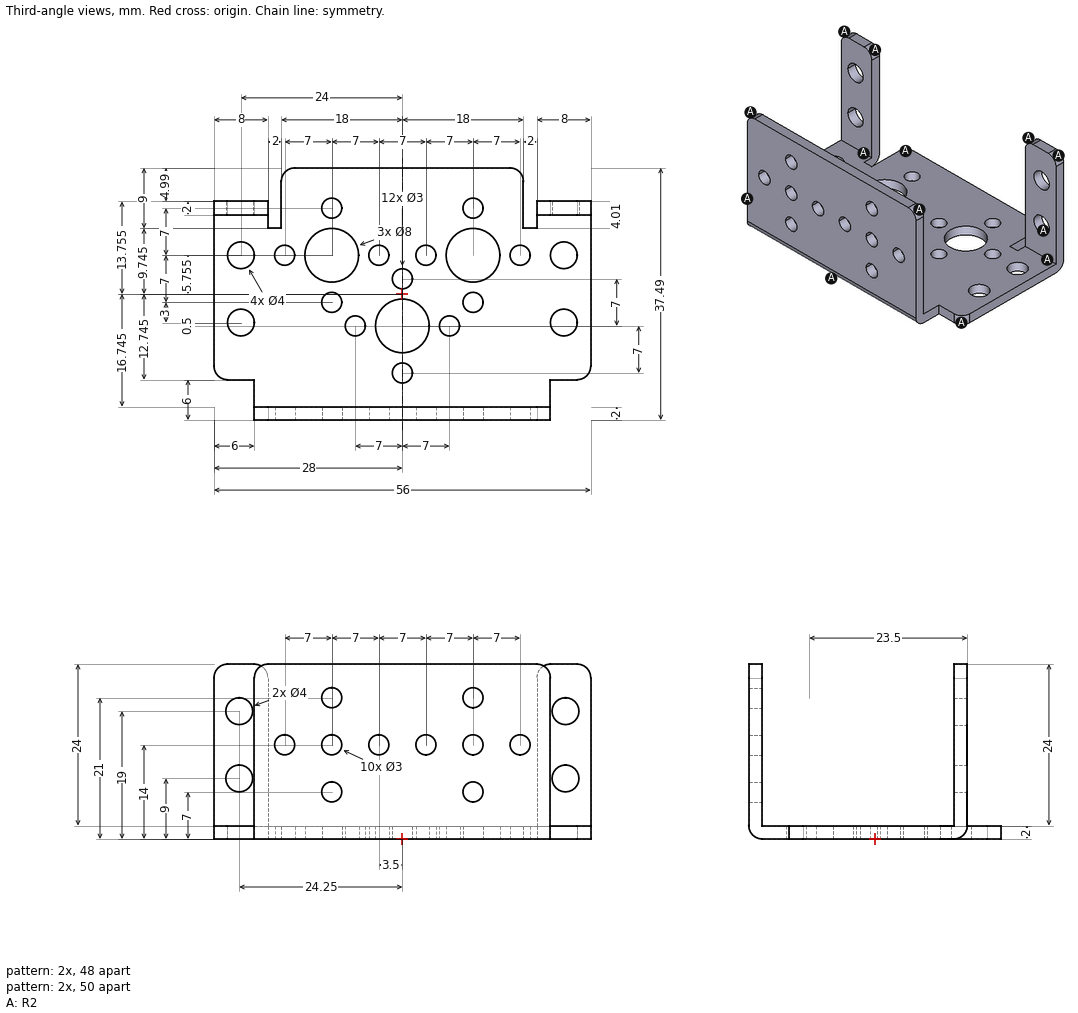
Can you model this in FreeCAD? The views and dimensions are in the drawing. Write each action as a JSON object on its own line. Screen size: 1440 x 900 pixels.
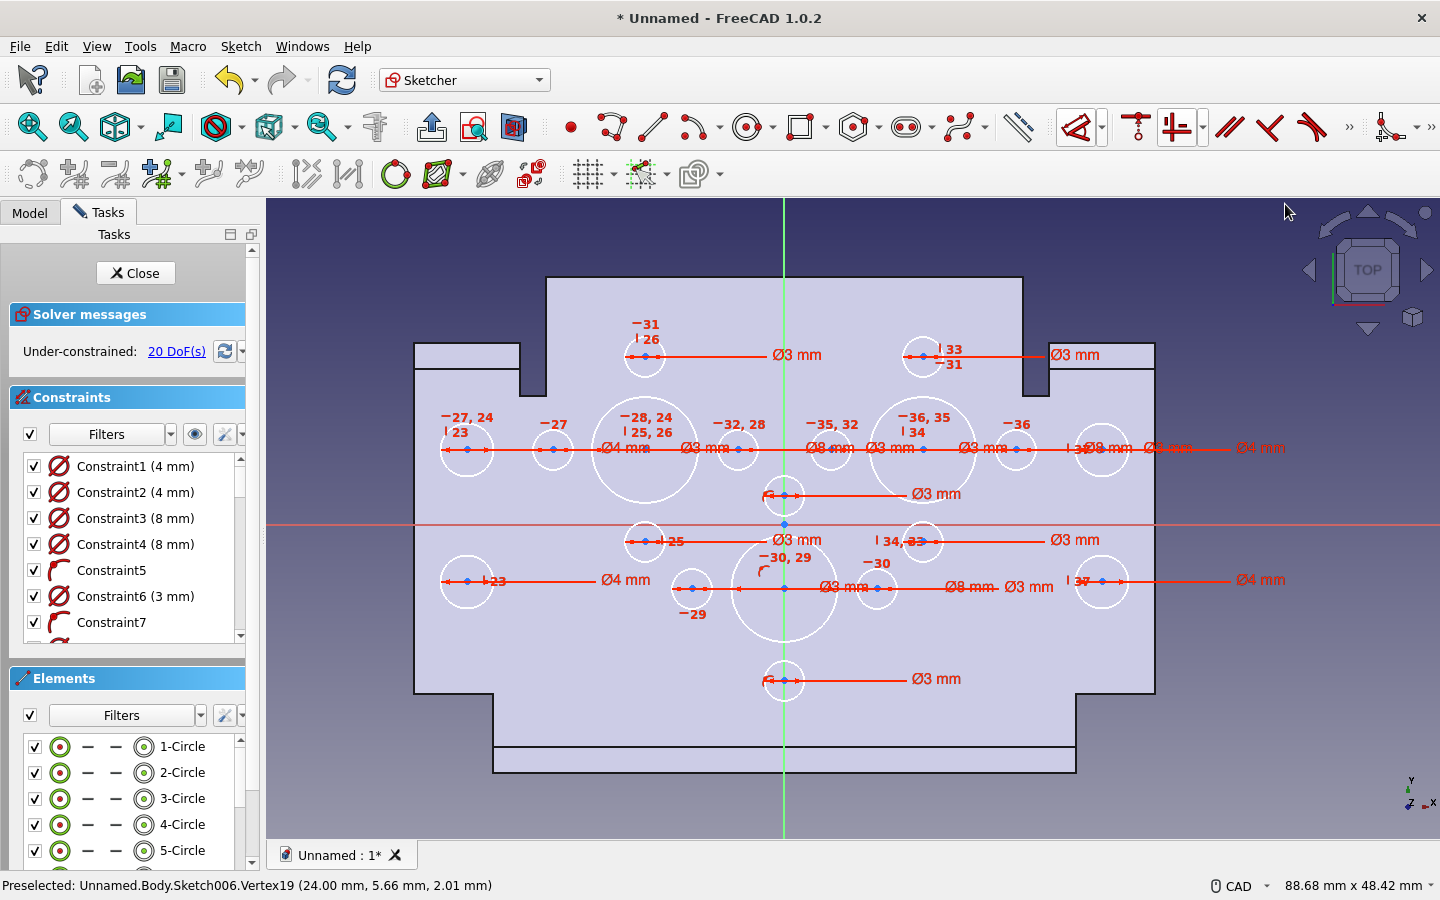
{"action": "left_click", "coordinate": [1016, 450]}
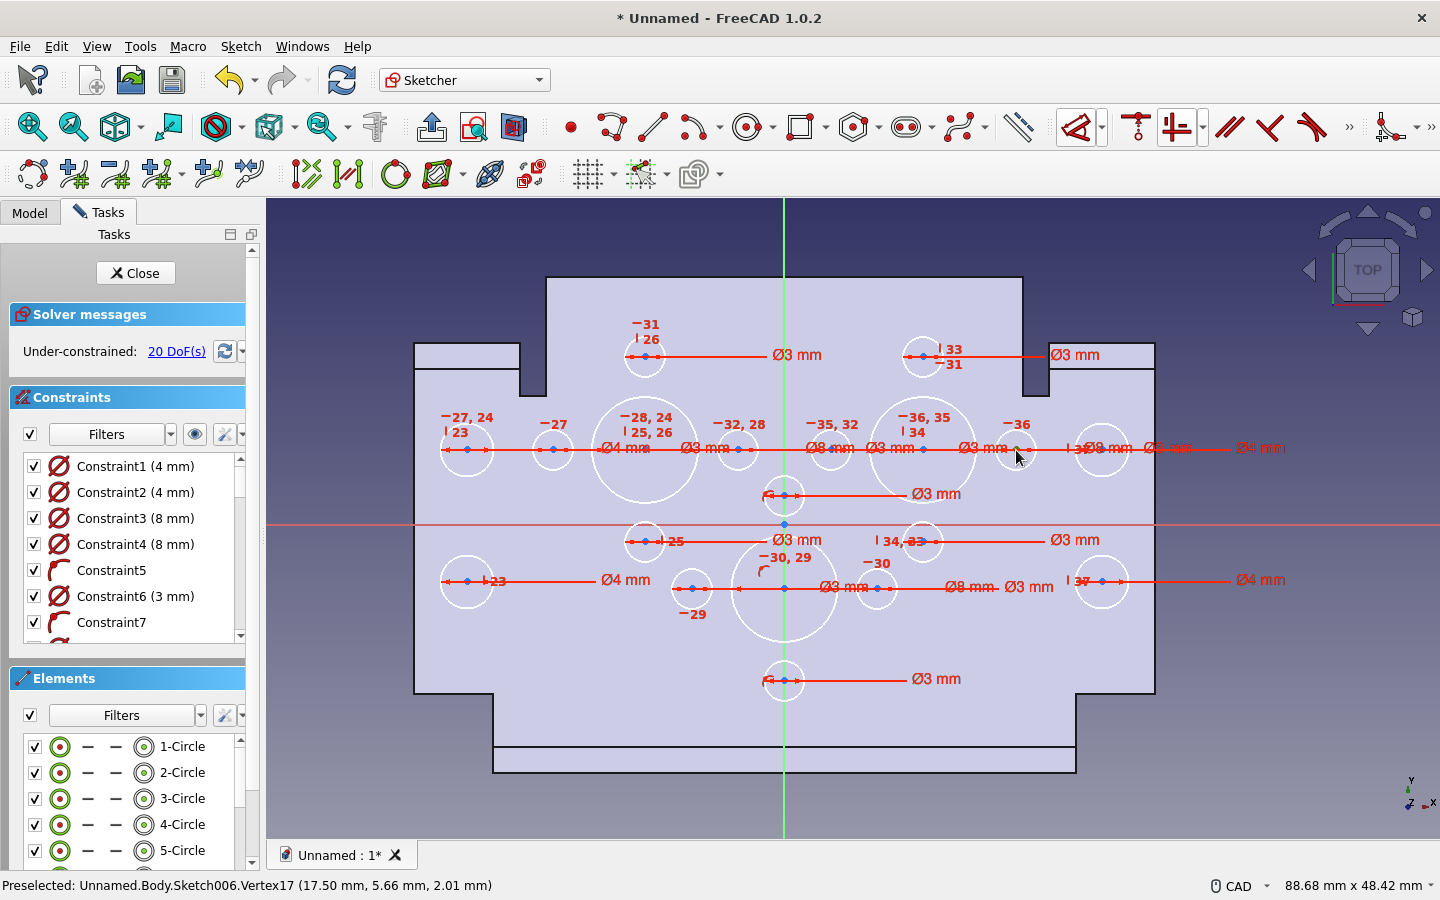
{"action": "left_click", "coordinate": [1102, 450]}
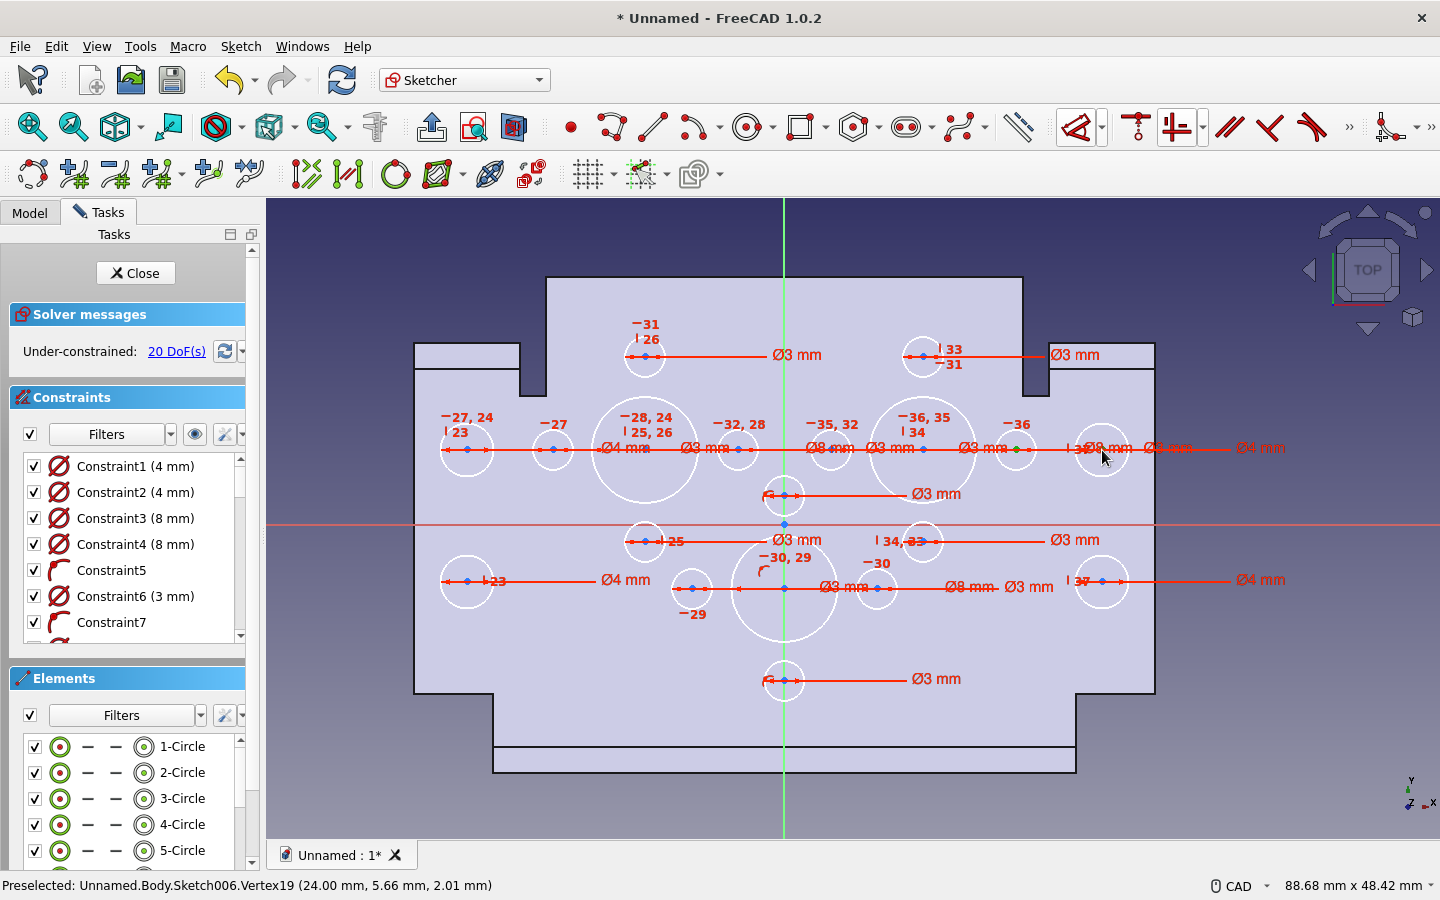
{"action": "left_click", "coordinate": [1202, 128]}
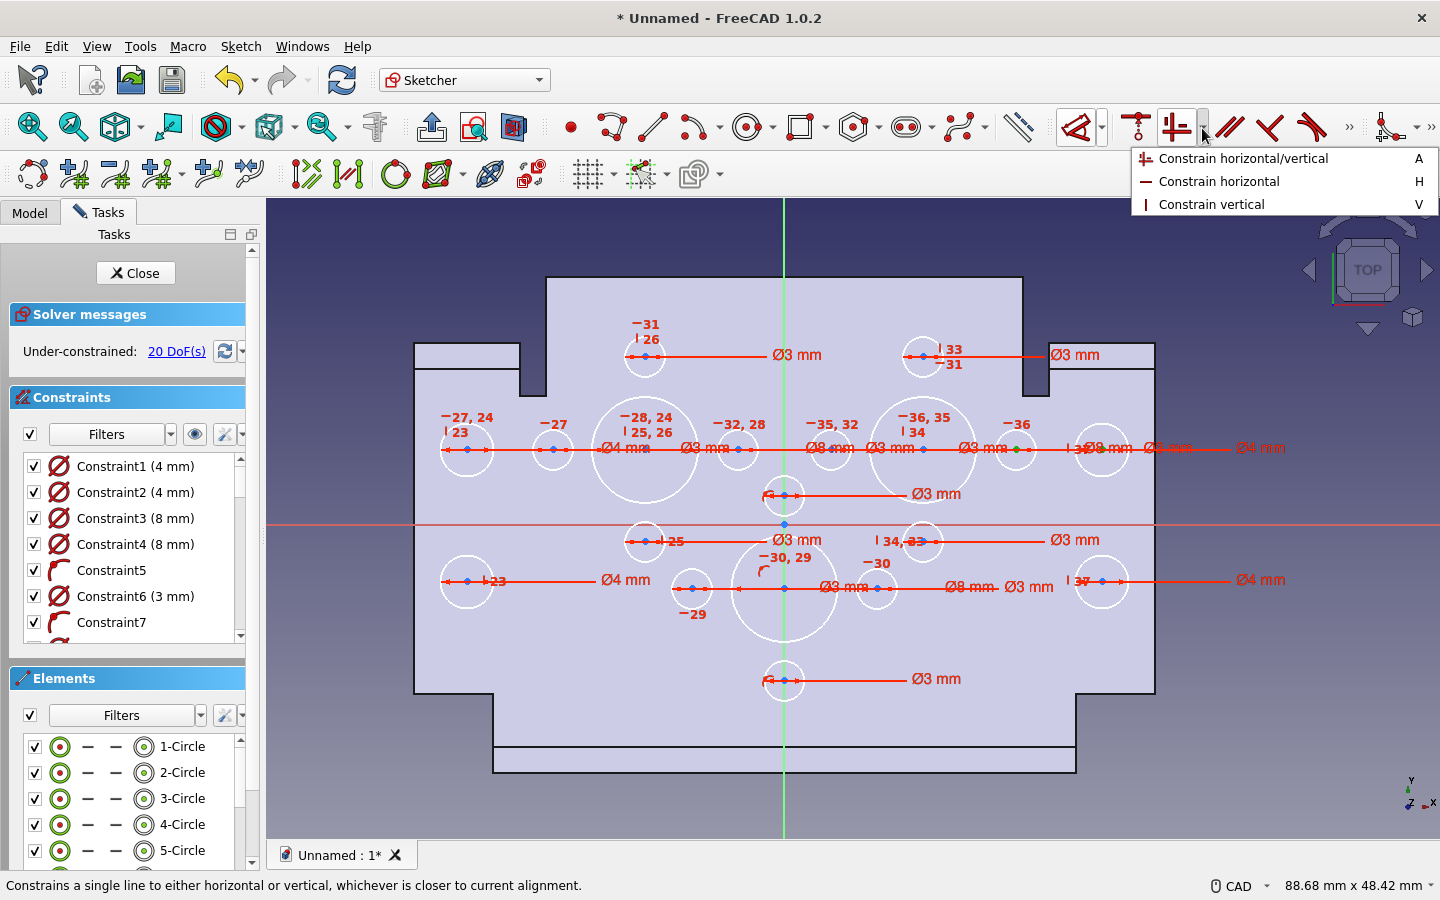
{"action": "left_click", "coordinate": [1285, 182]}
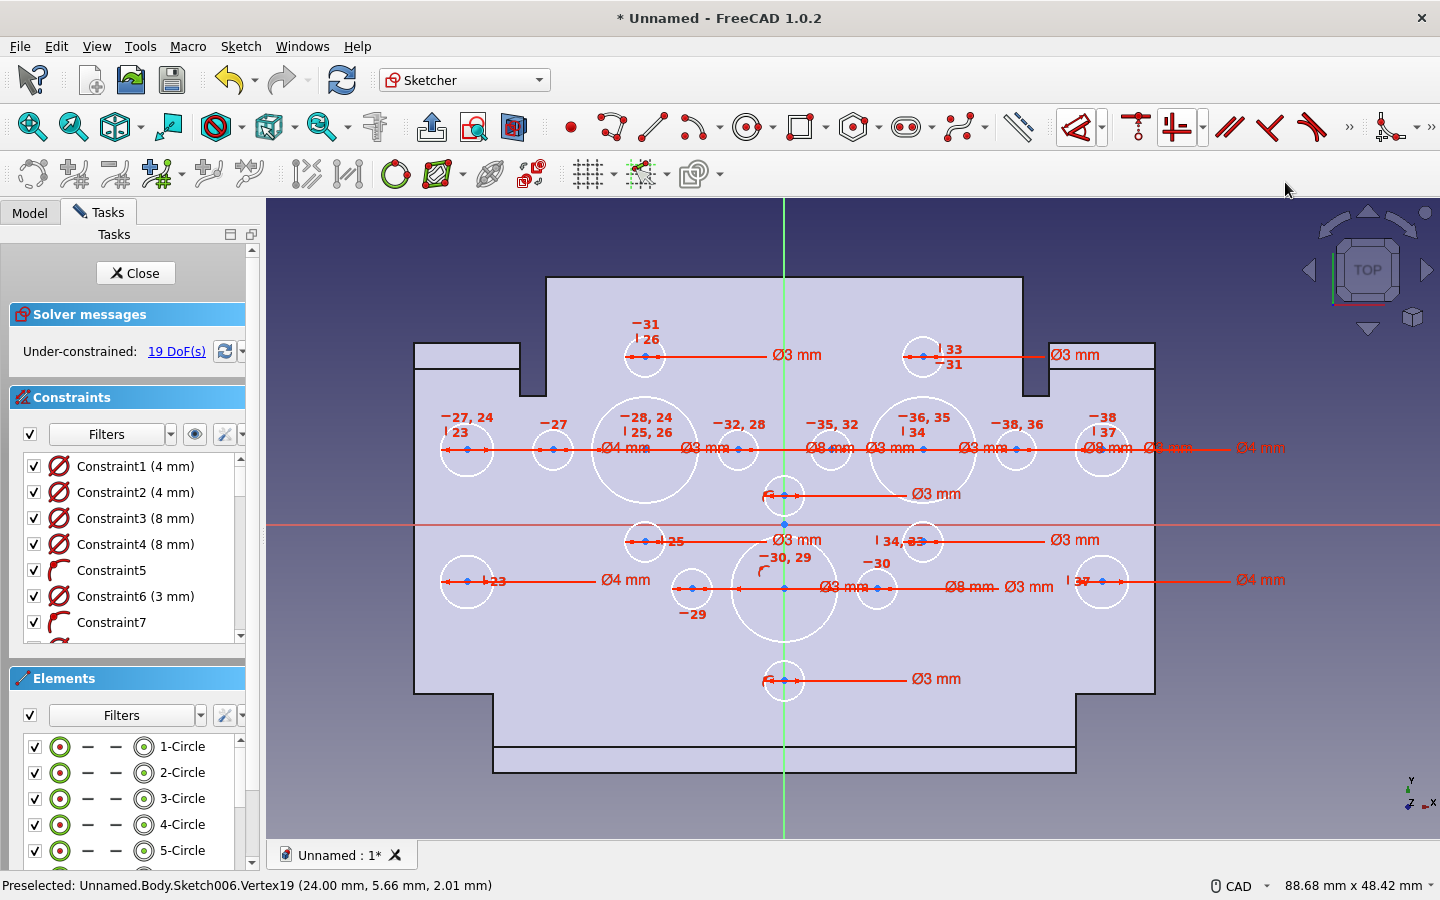
{"action": "left_click", "coordinate": [645, 542]}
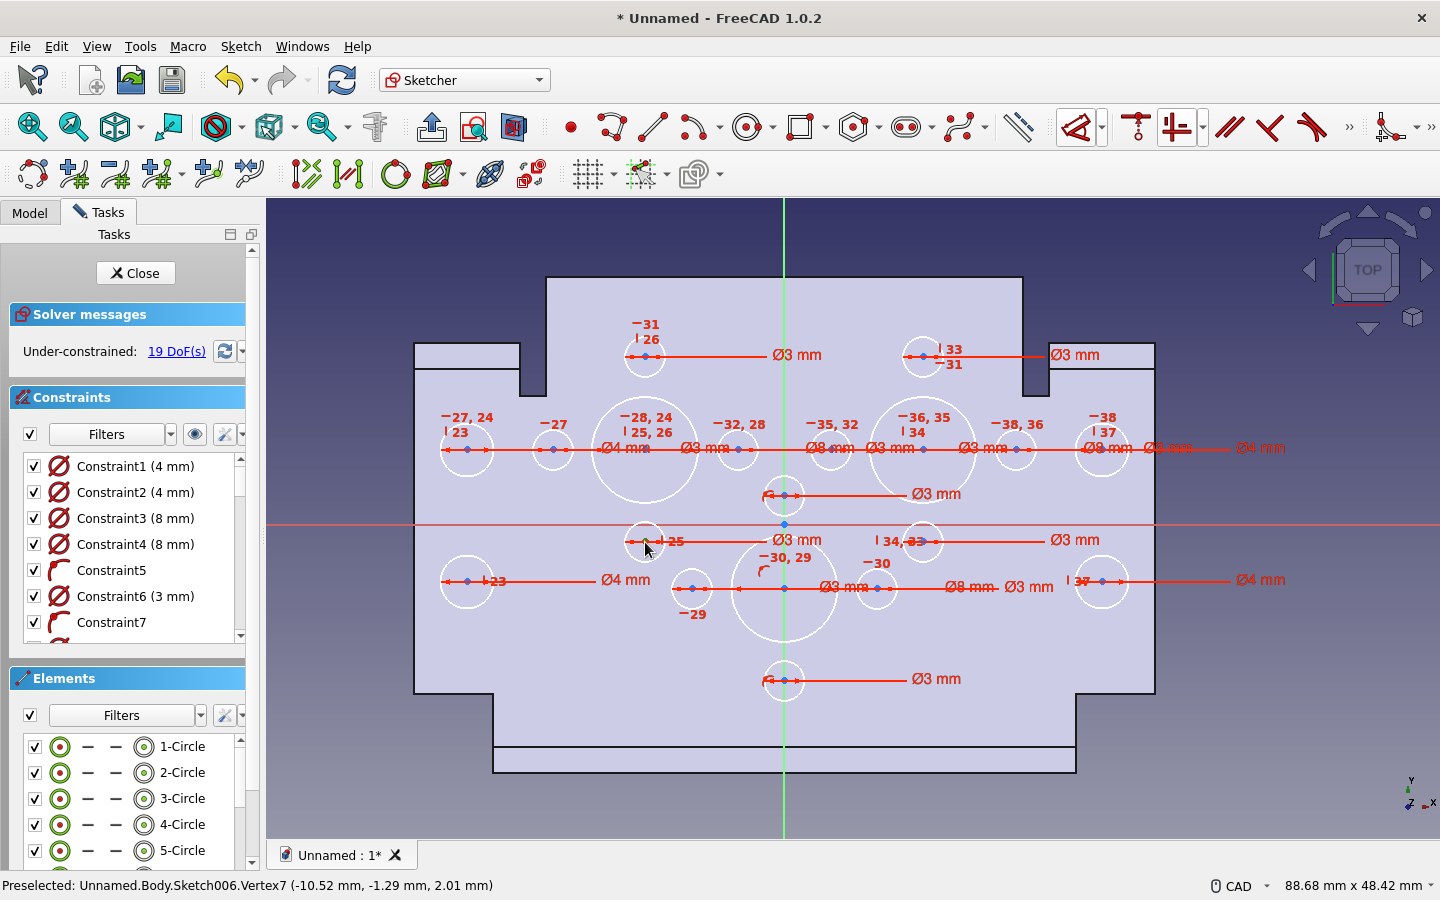
{"action": "left_click", "coordinate": [923, 542]}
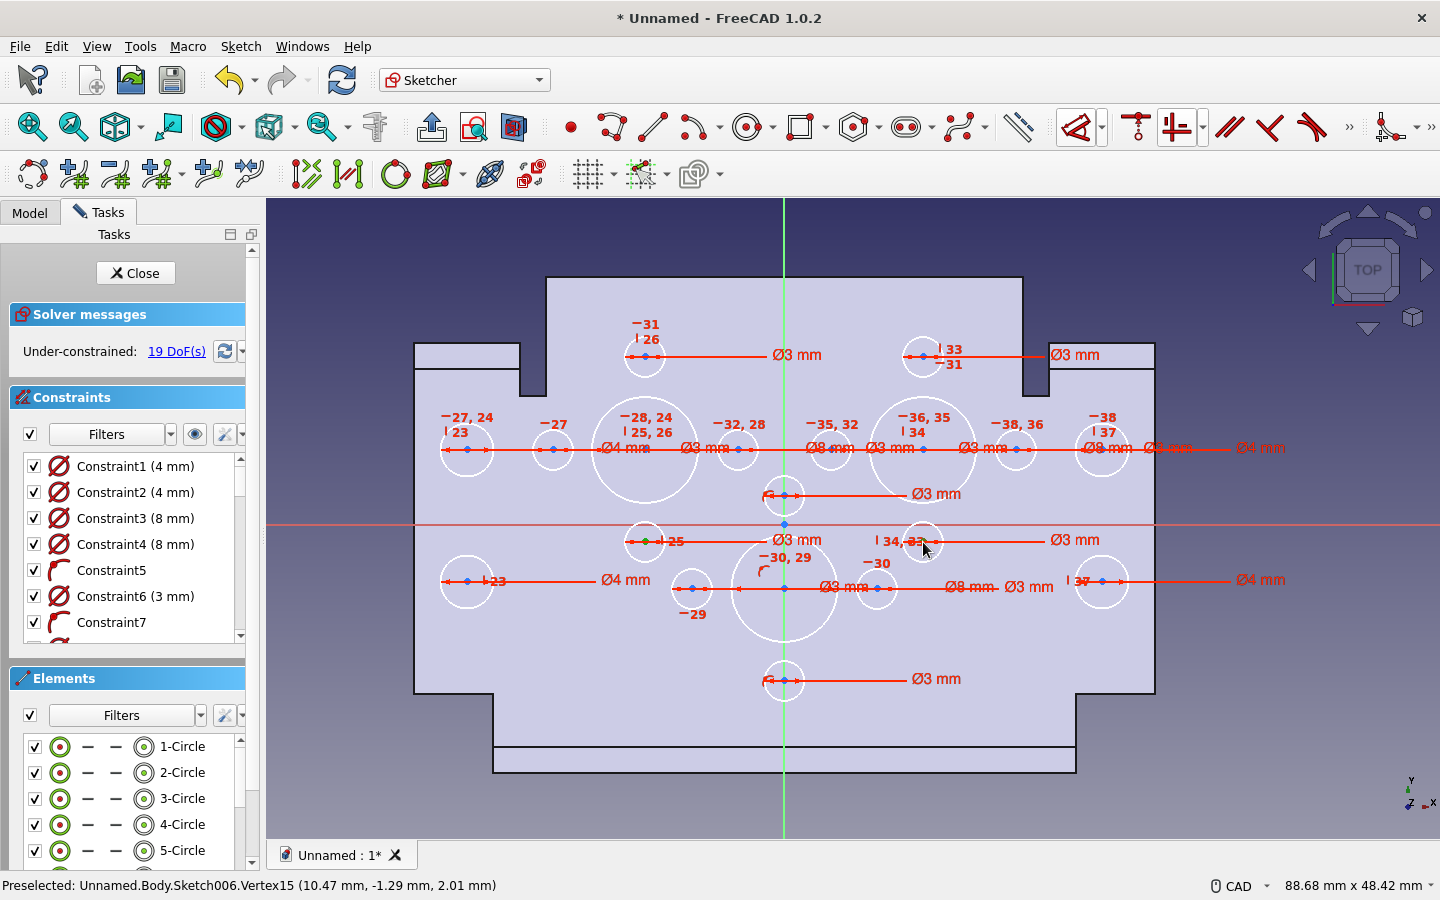
{"action": "left_click", "coordinate": [784, 769]}